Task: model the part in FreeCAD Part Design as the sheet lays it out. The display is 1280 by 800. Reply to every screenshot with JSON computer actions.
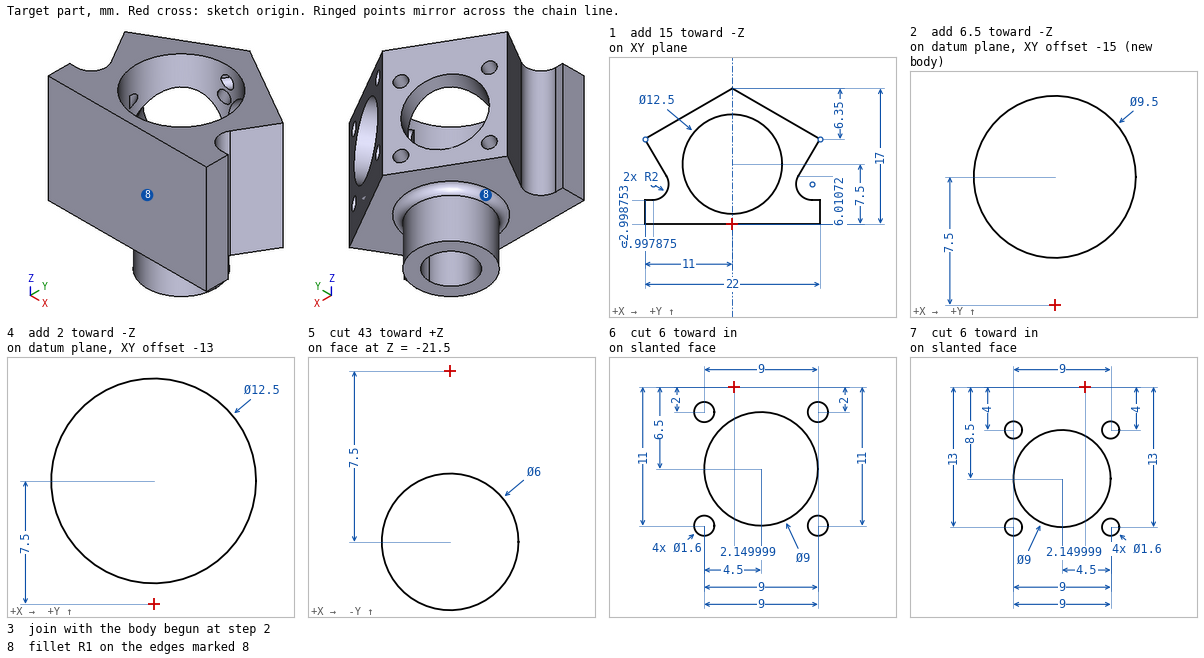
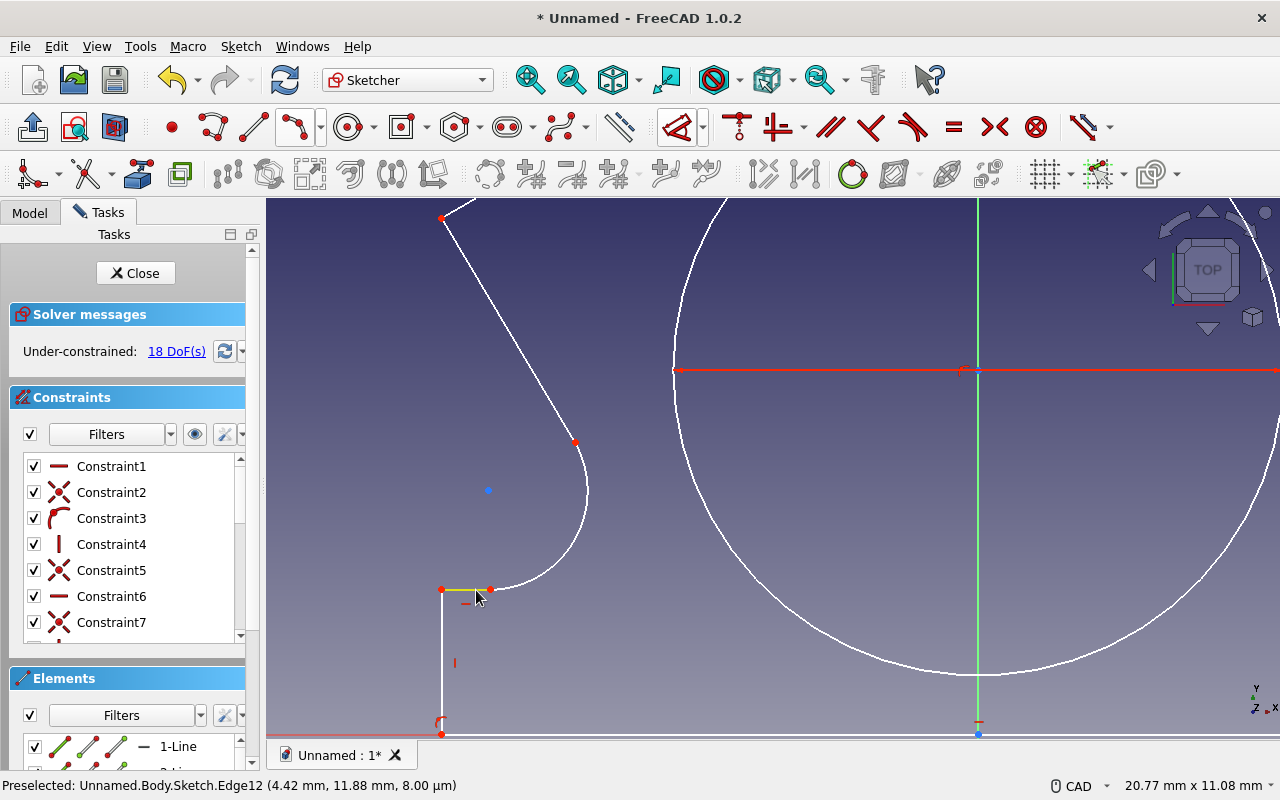
{"action": "left_click", "coordinate": [476, 590]}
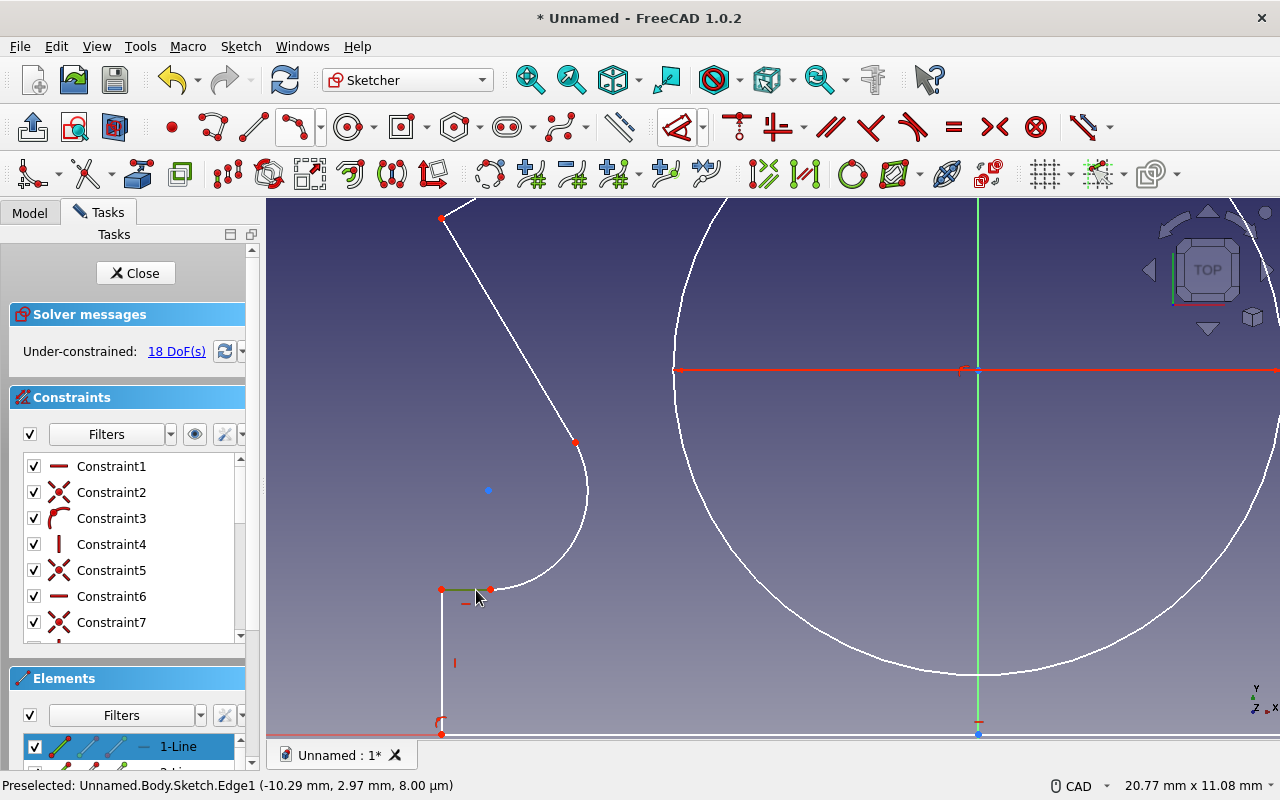
{"action": "left_click", "coordinate": [548, 570]}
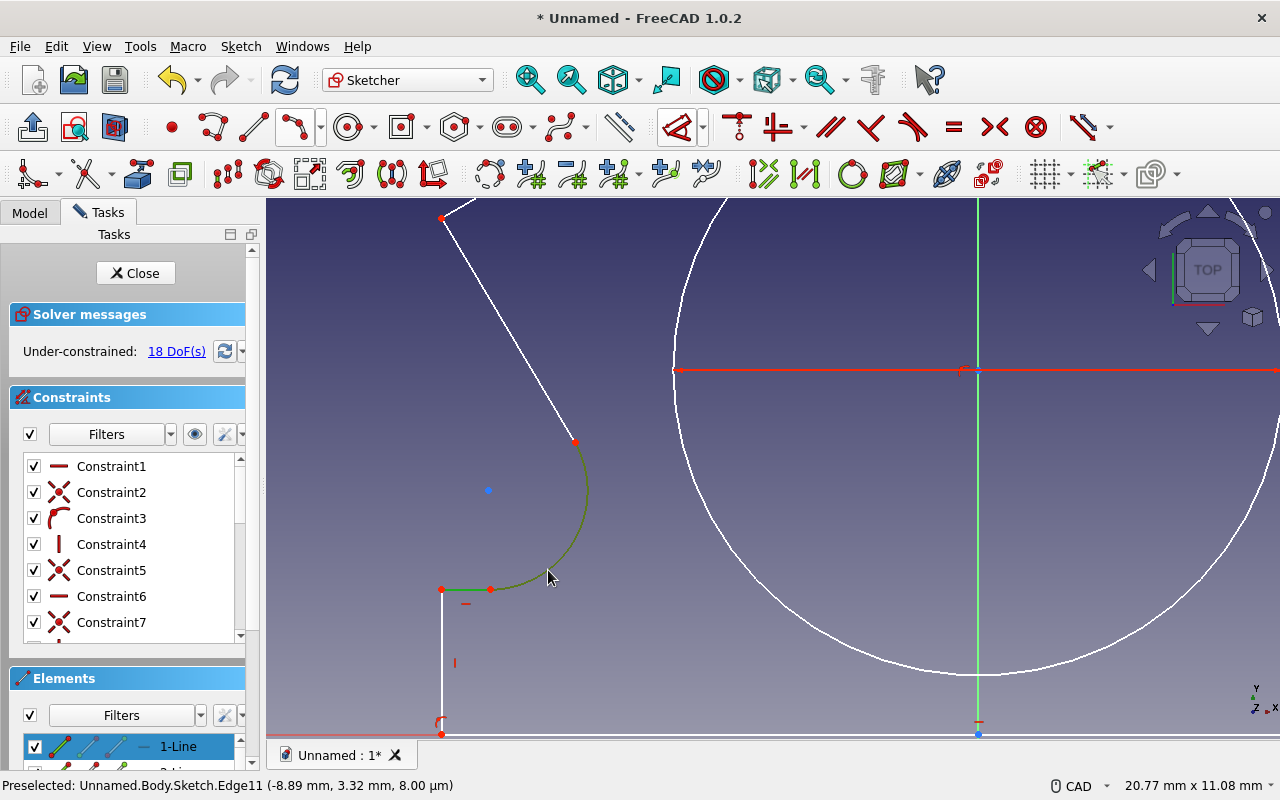
{"action": "left_click", "coordinate": [913, 128]}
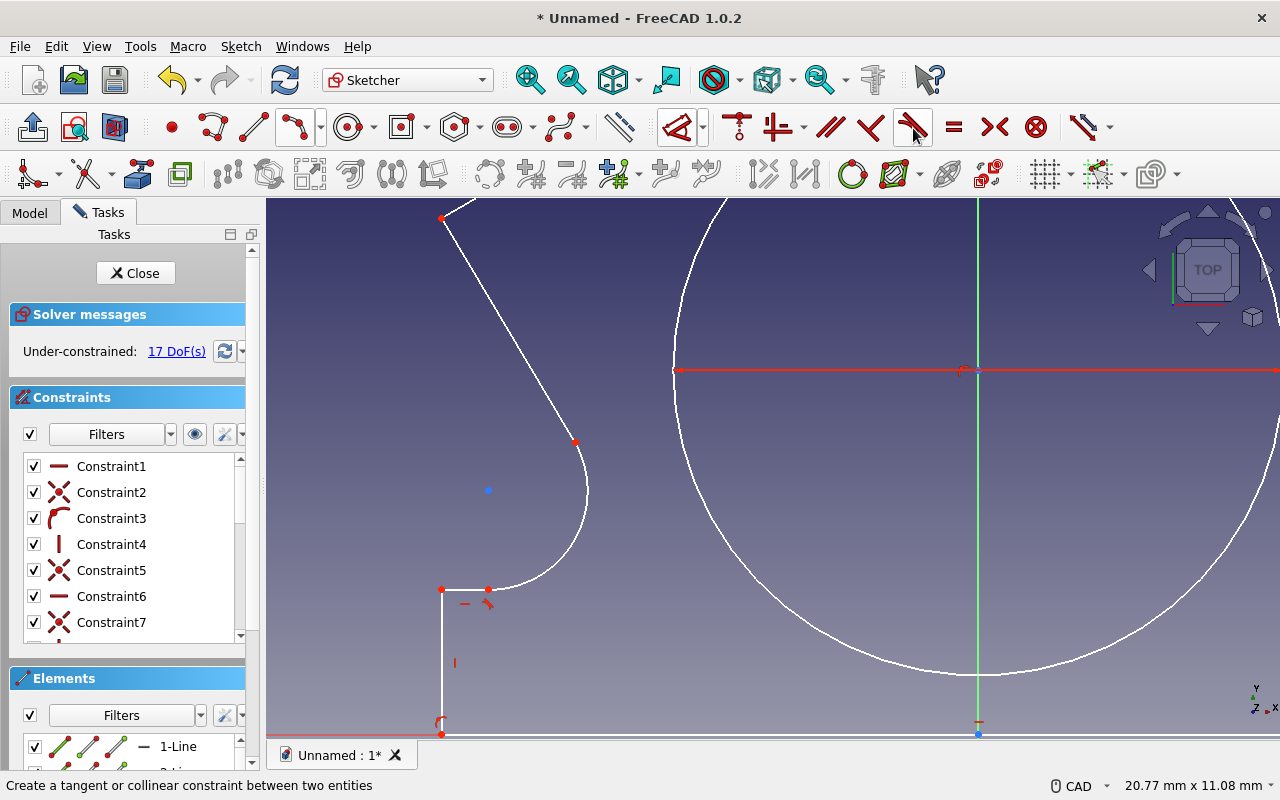
{"action": "scroll", "coordinate": [481, 590], "scroll_direction": "down", "scroll_amount": 4}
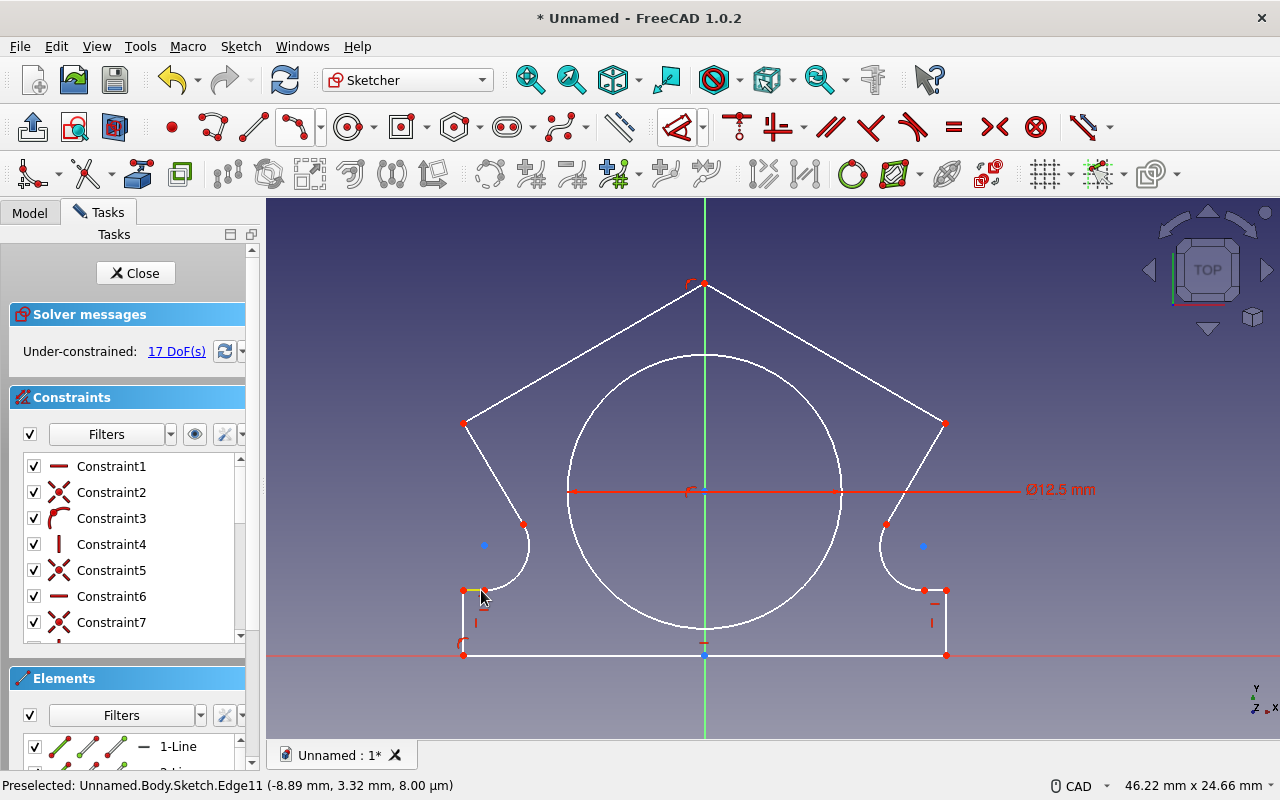
{"action": "scroll", "coordinate": [940, 590], "scroll_direction": "up", "scroll_amount": 4}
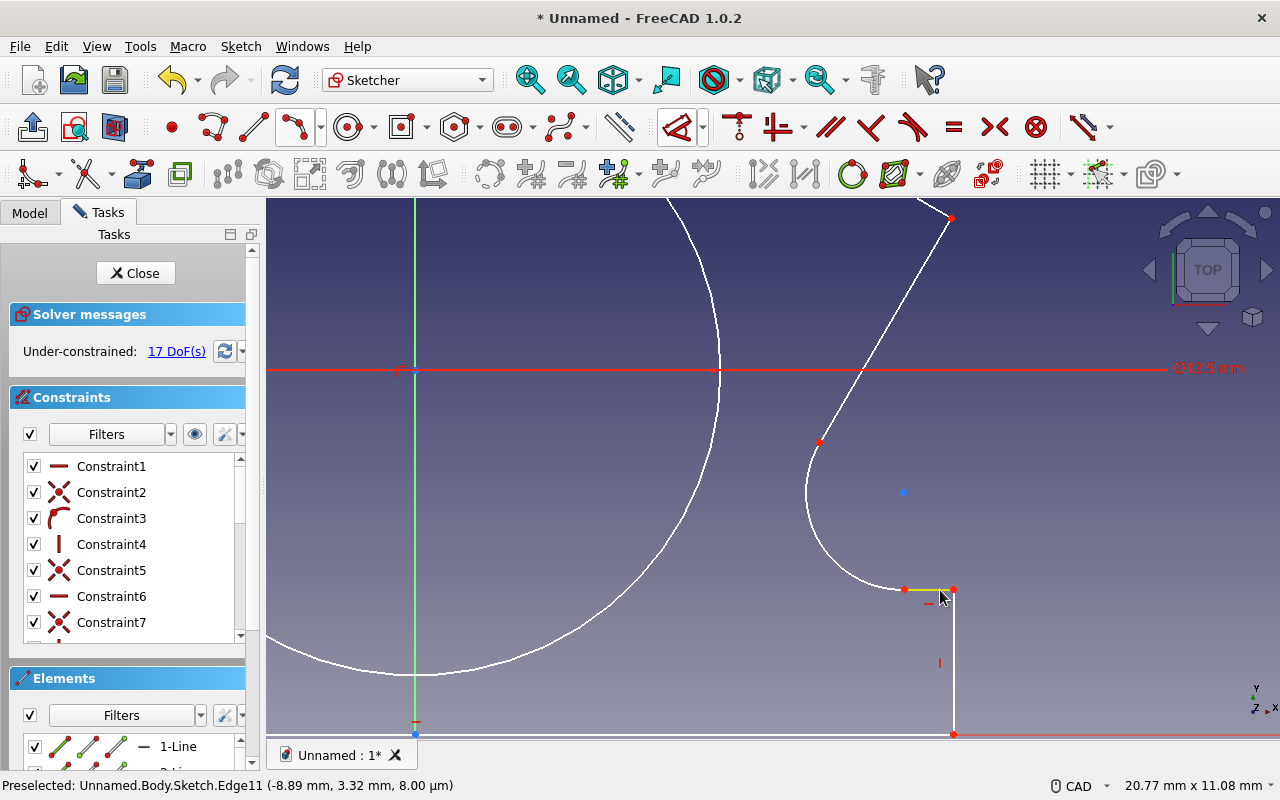
{"action": "left_click", "coordinate": [939, 590]}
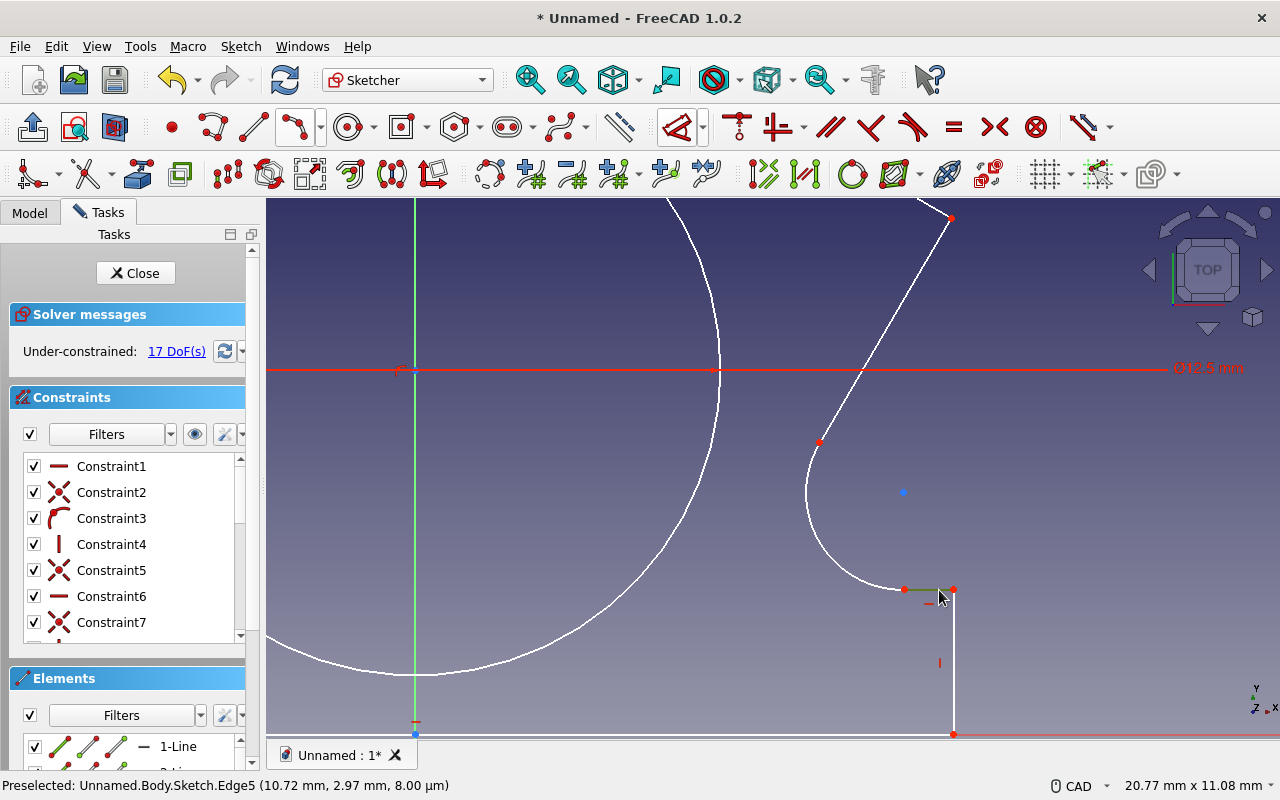
{"action": "left_click", "coordinate": [807, 502]}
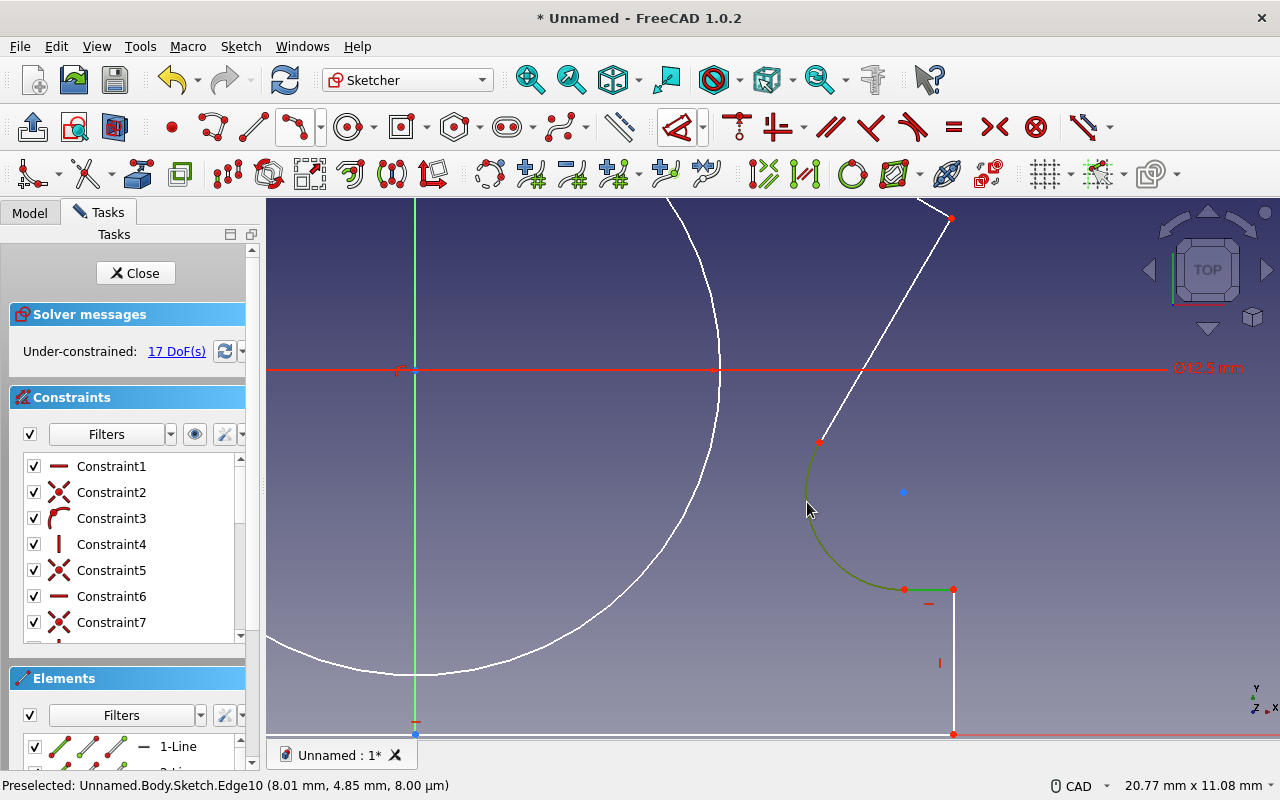
{"action": "left_click", "coordinate": [913, 128]}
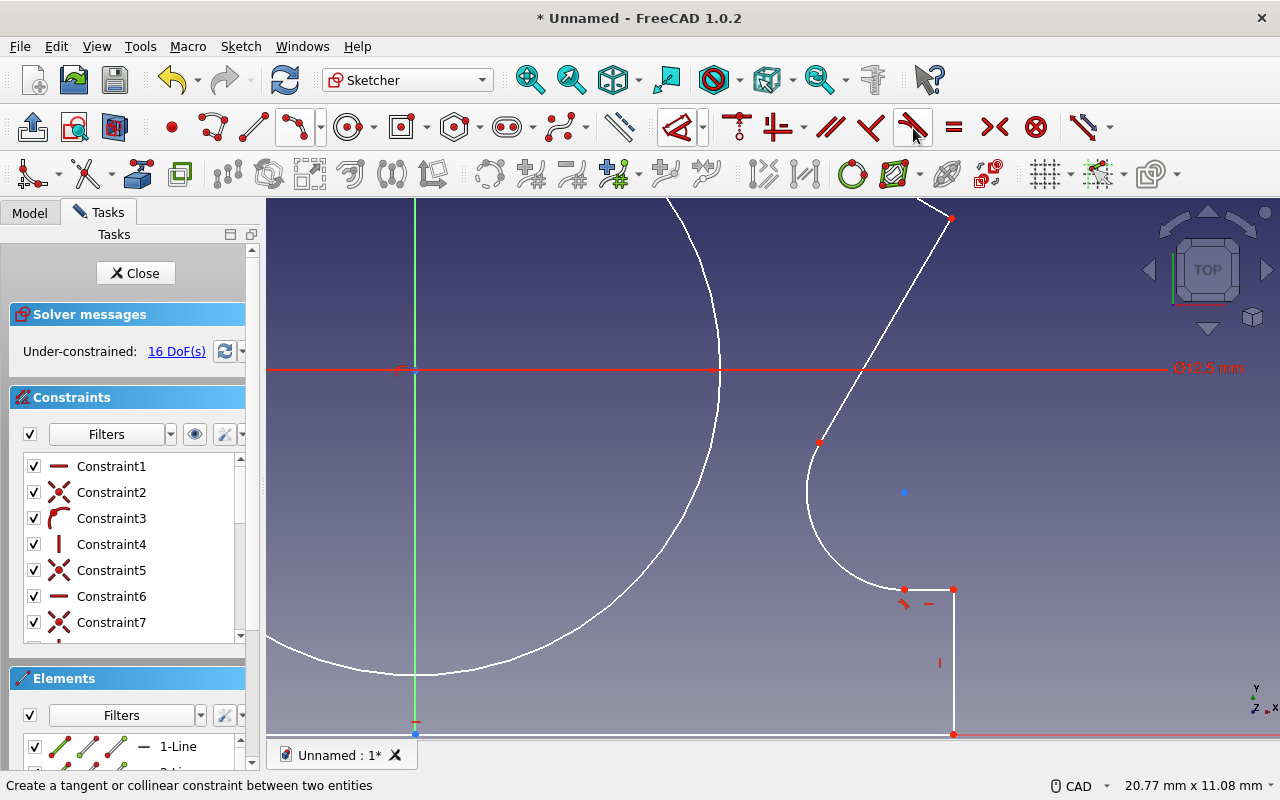
{"action": "left_click", "coordinate": [859, 376]}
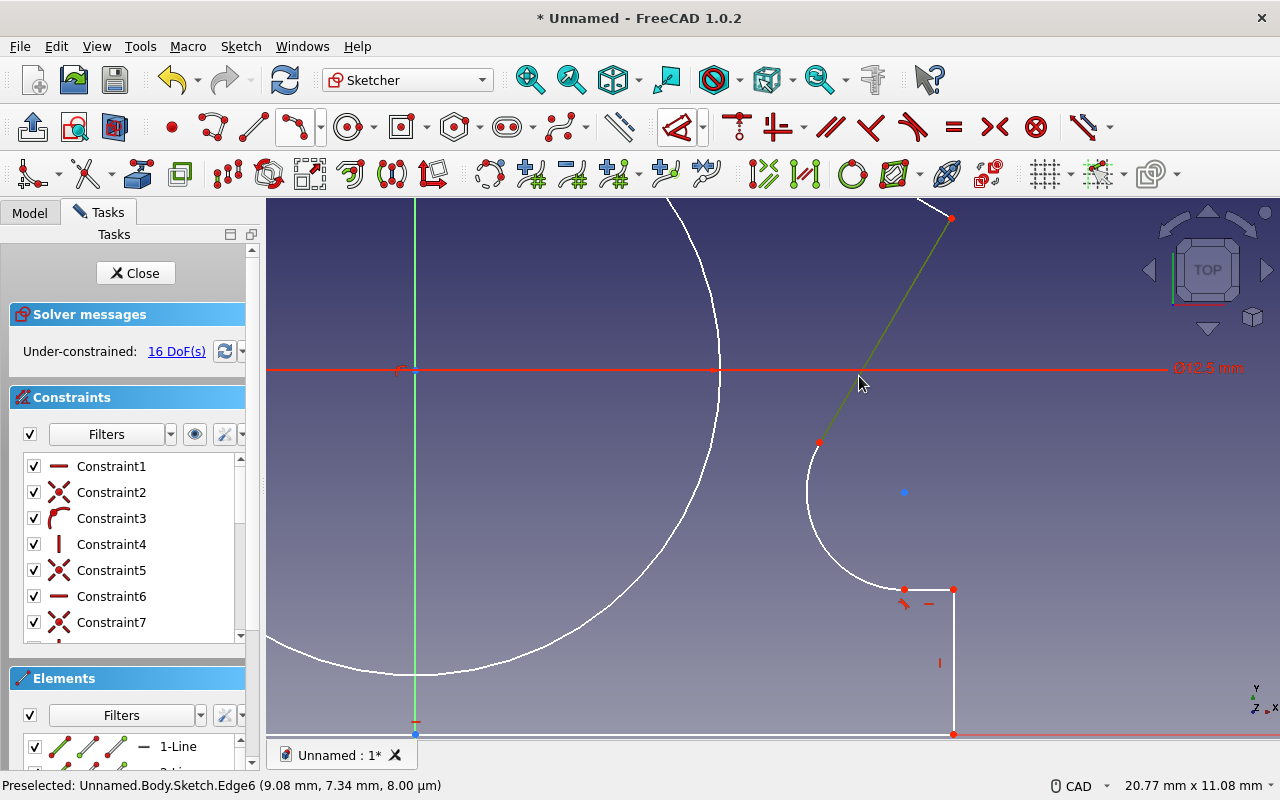
{"action": "left_click", "coordinate": [807, 502]}